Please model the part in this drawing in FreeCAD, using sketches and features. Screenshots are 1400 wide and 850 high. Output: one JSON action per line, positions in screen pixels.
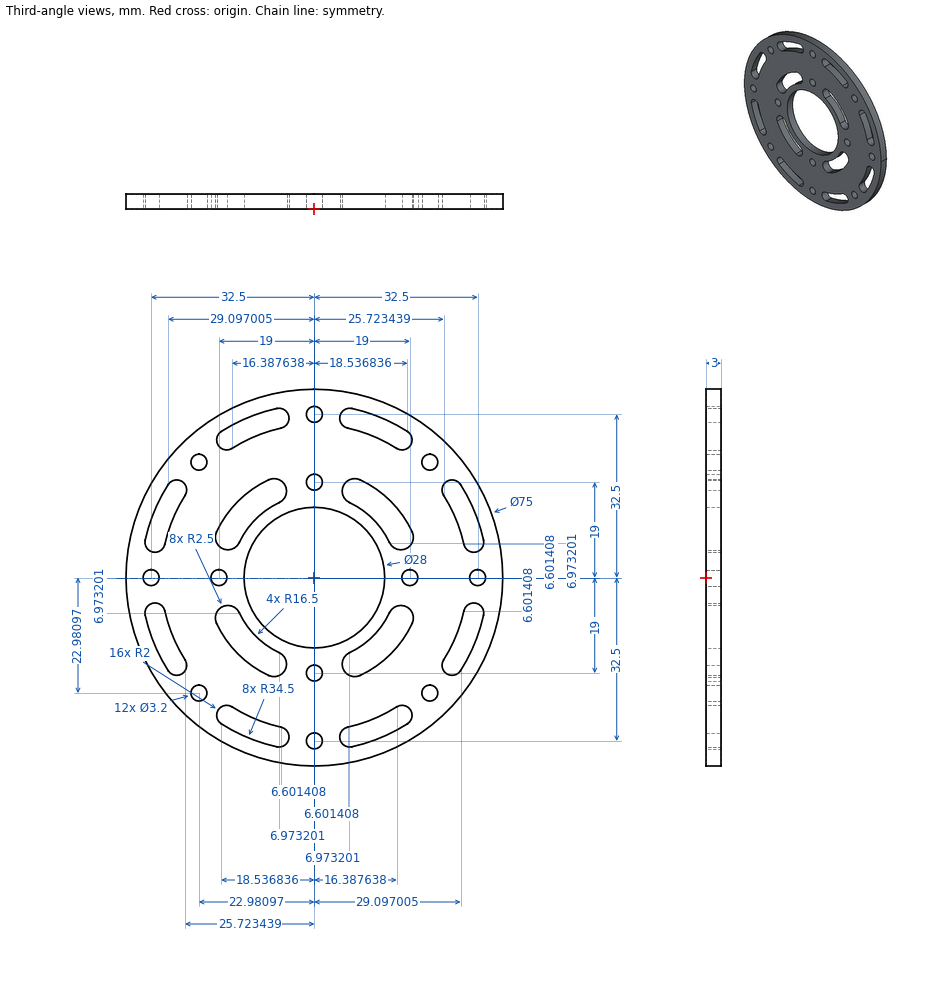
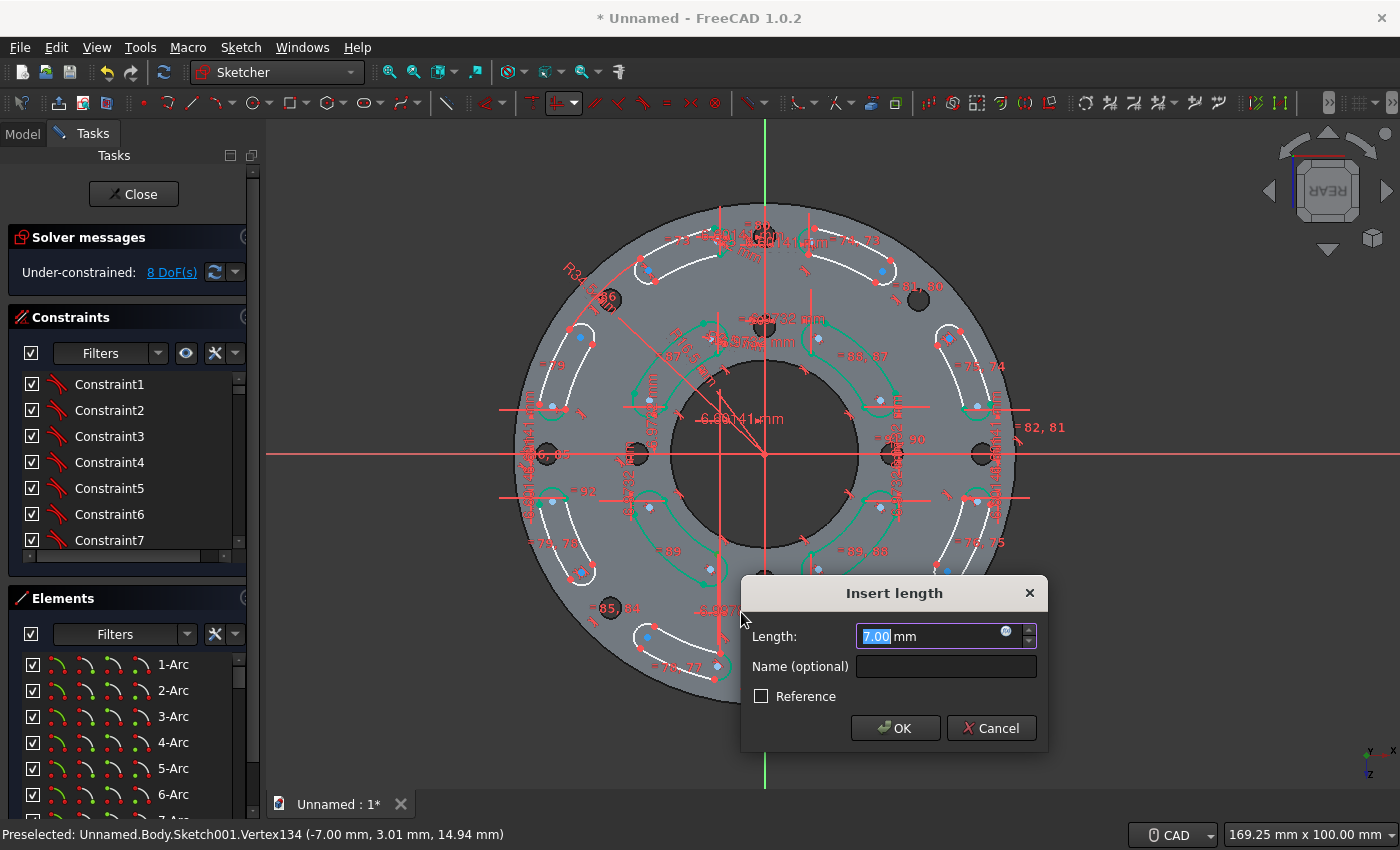
{"action": "type", "text": "6.973201"}
{"action": "key", "text": "Return"}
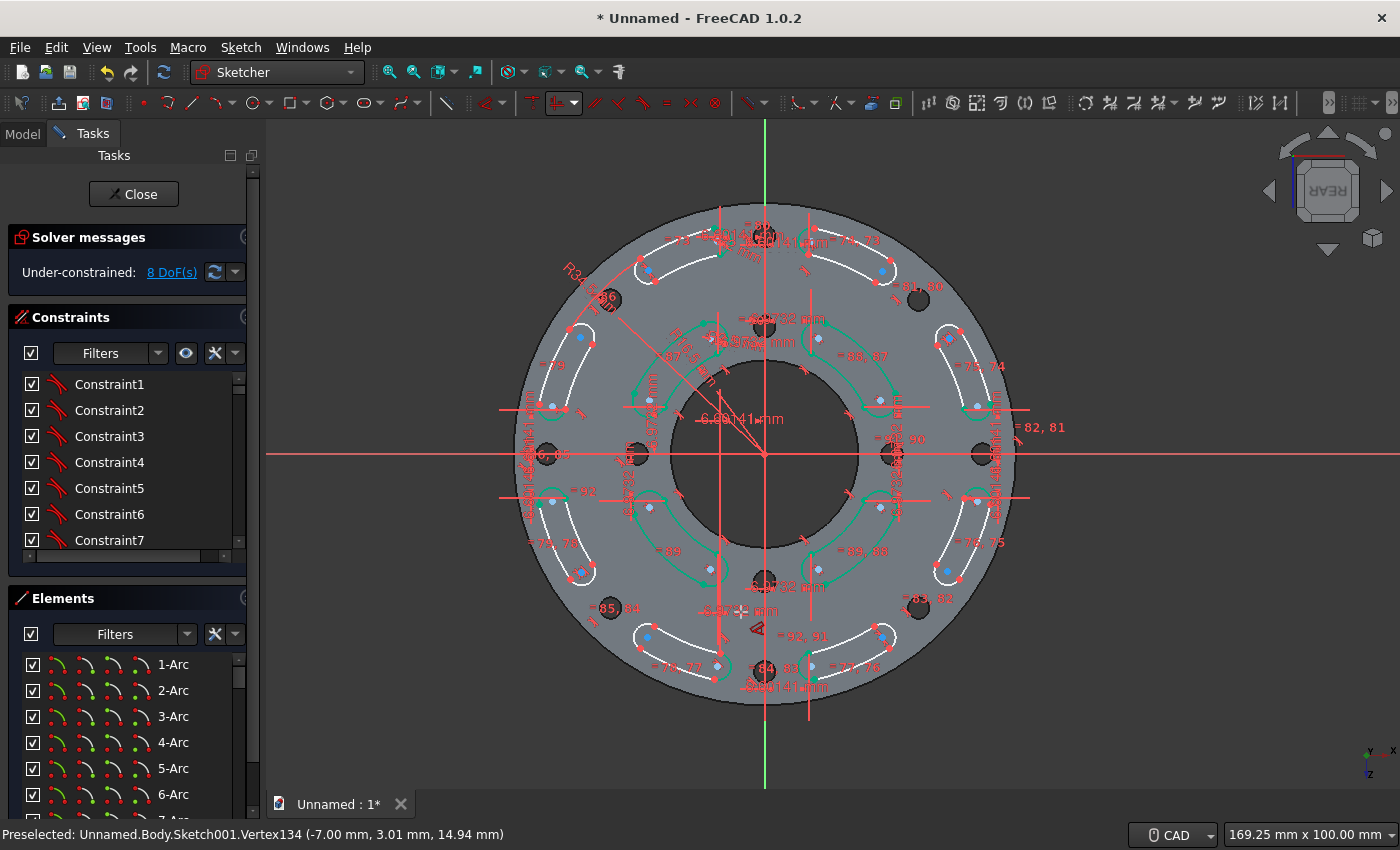
{"action": "left_click", "coordinate": [641, 259]}
{"action": "left_click", "coordinate": [659, 225]}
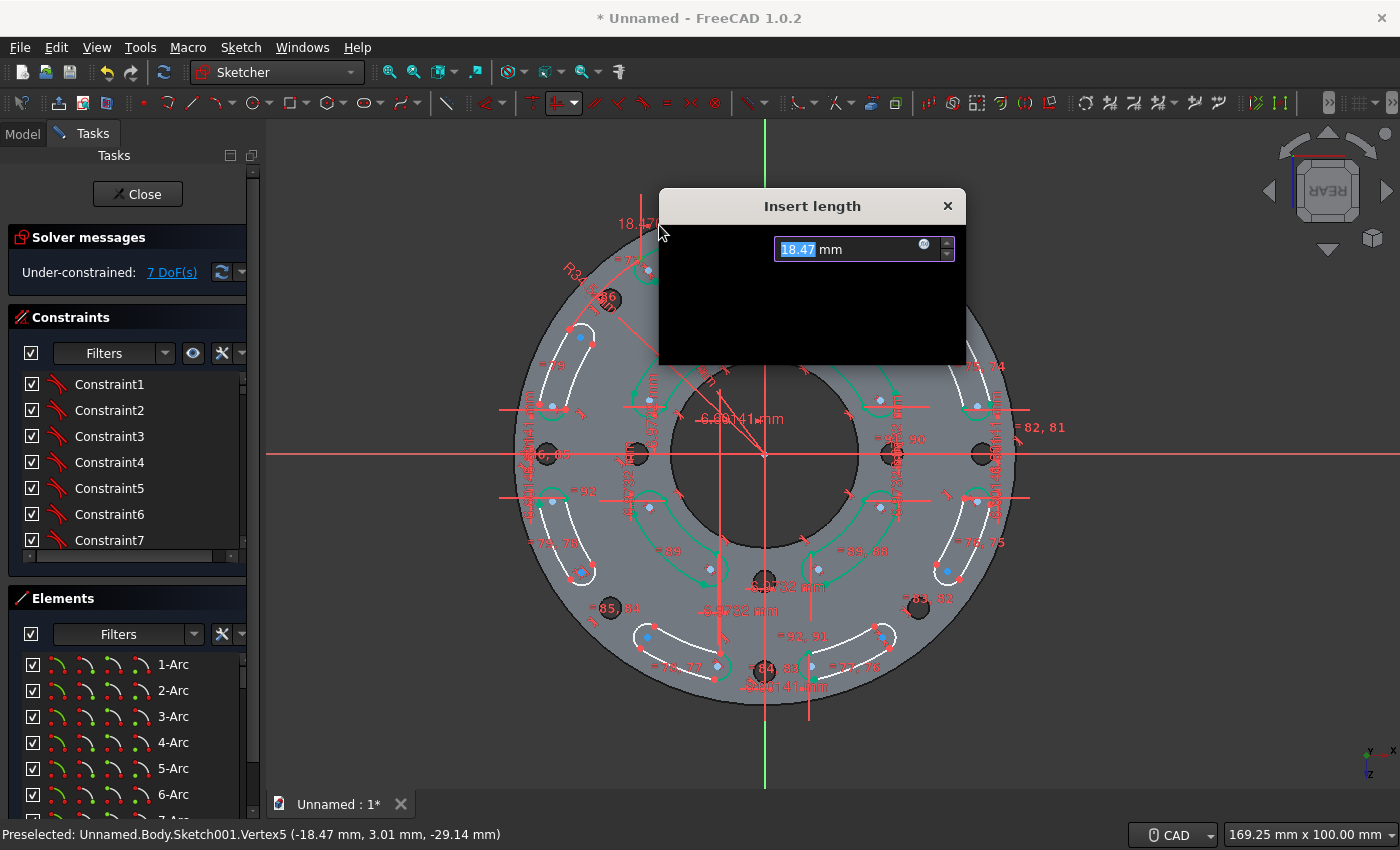
{"action": "type", "text": "18.536836"}
{"action": "key", "text": "Return"}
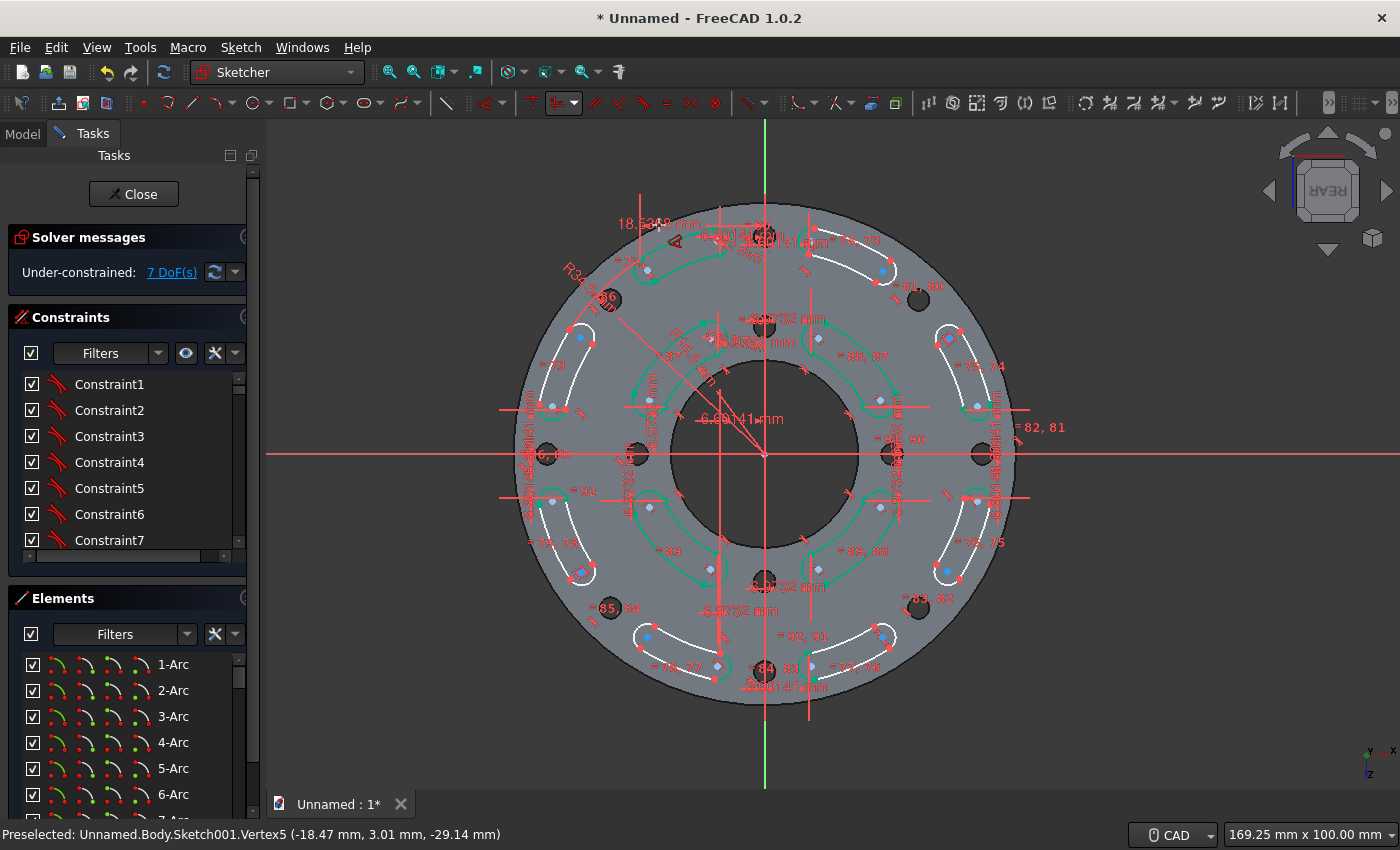
{"action": "left_click", "coordinate": [876, 283]}
{"action": "left_click", "coordinate": [820, 488]}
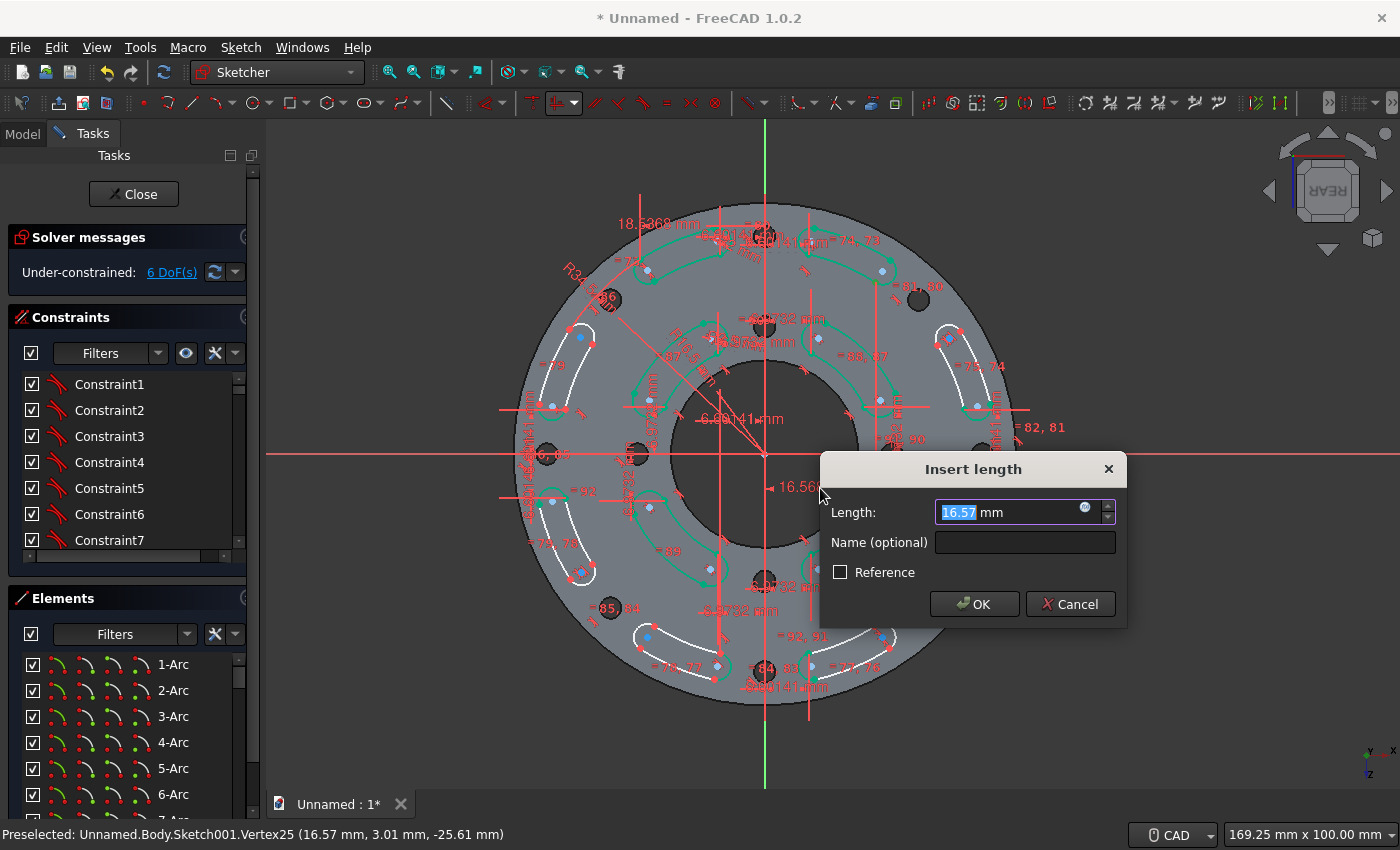
{"action": "type", "text": "16.387638"}
{"action": "key", "text": "Return"}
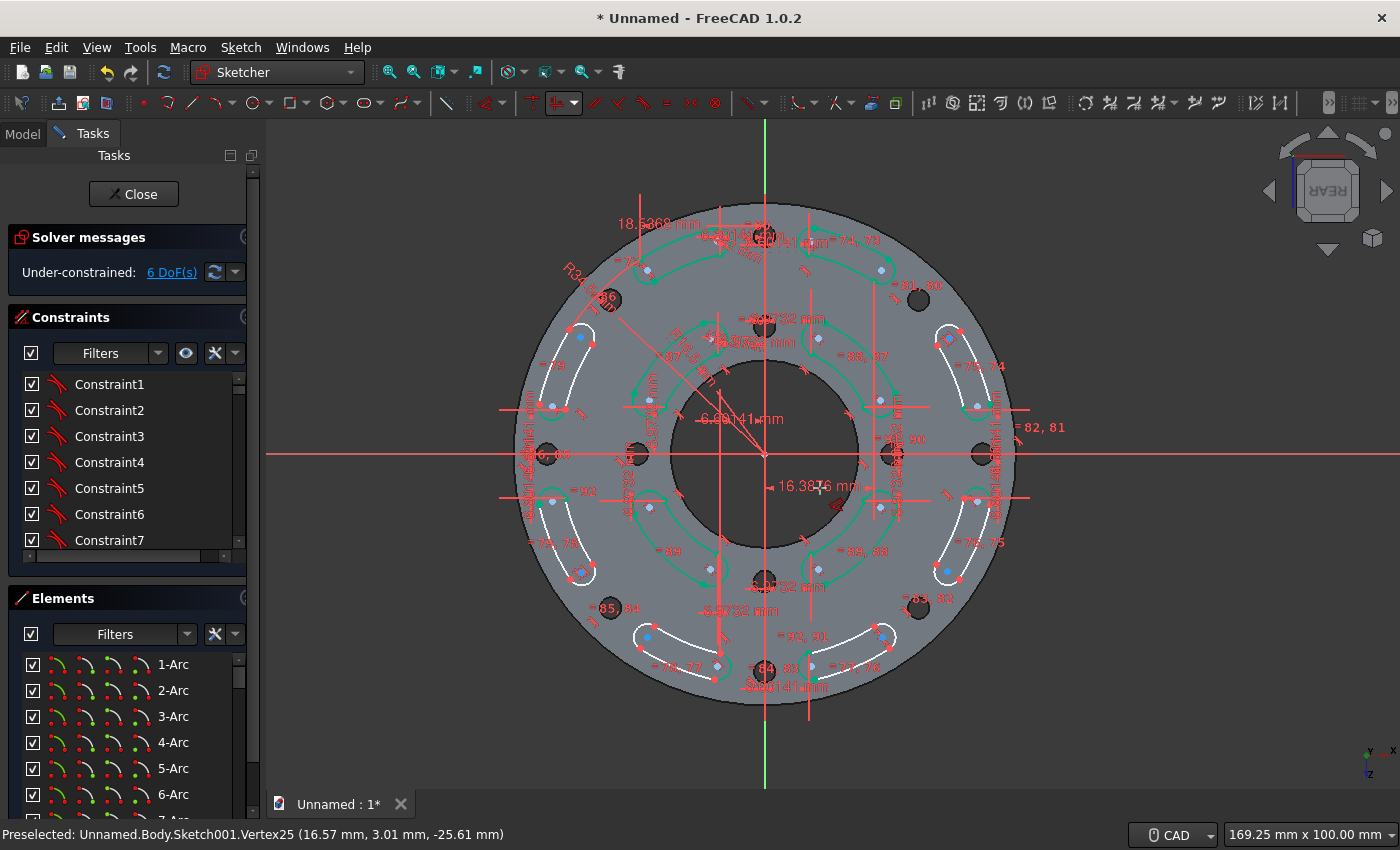
{"action": "left_click", "coordinate": [960, 331]}
{"action": "left_click", "coordinate": [863, 297]}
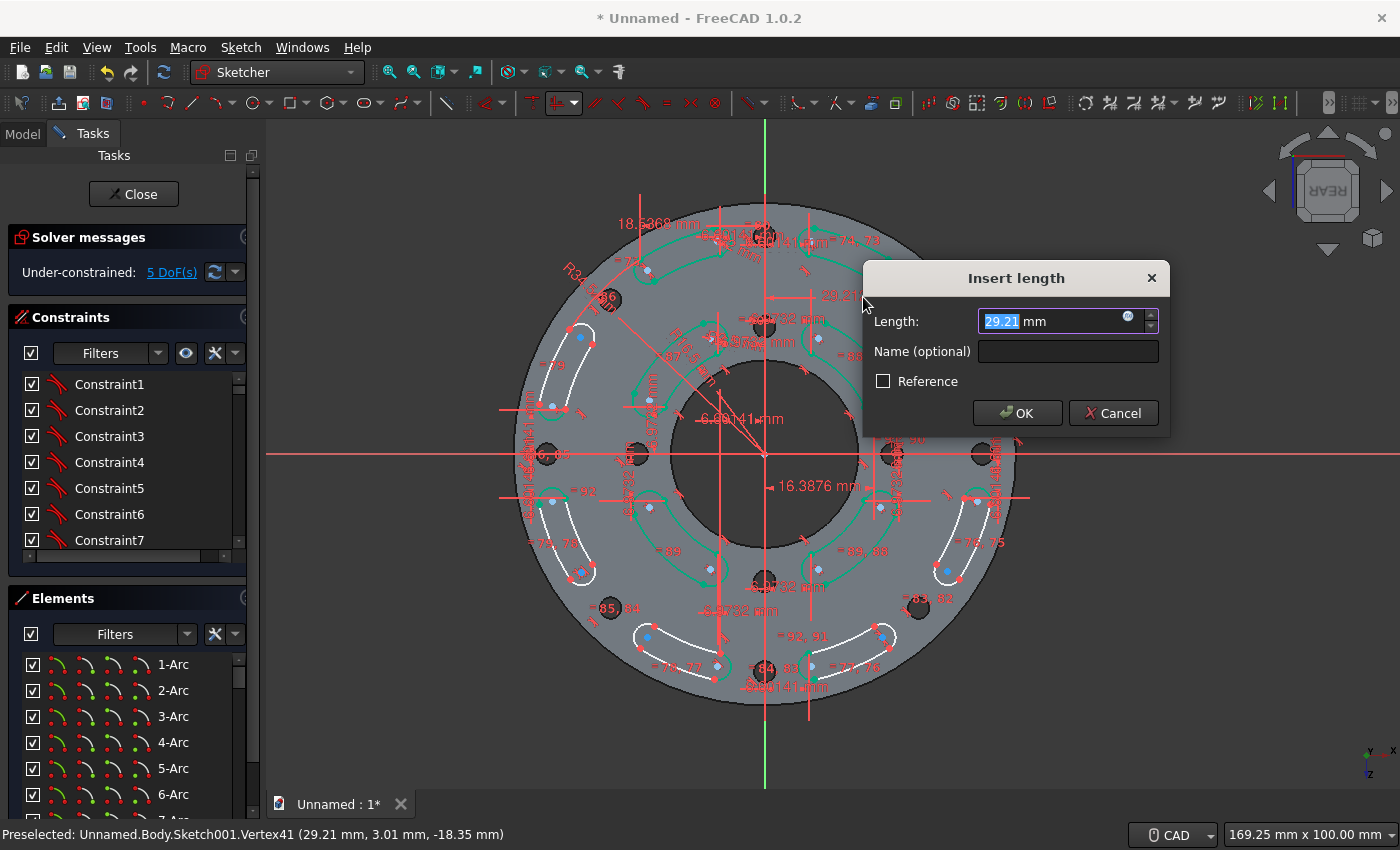
{"action": "type", "text": "29.097005"}
{"action": "key", "text": "Return"}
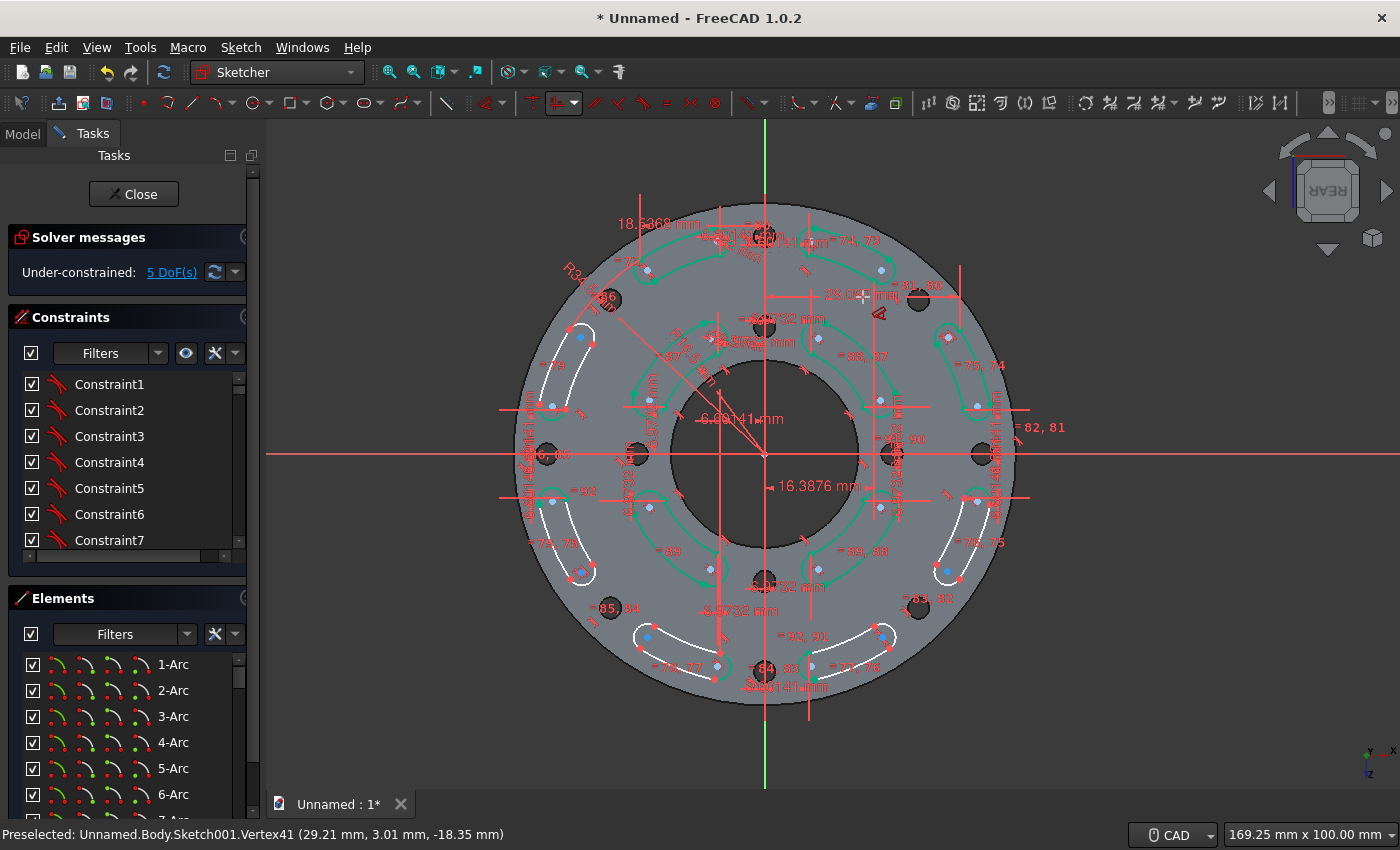
{"action": "left_click", "coordinate": [937, 565]}
{"action": "left_click", "coordinate": [890, 599]}